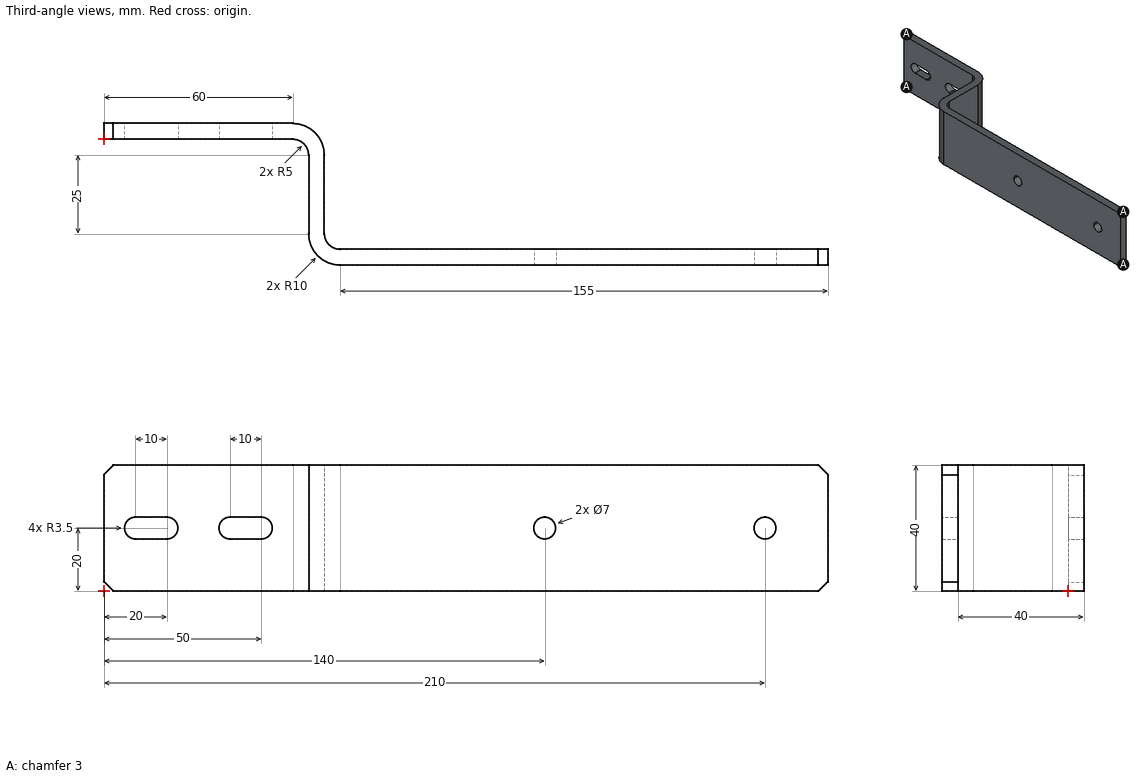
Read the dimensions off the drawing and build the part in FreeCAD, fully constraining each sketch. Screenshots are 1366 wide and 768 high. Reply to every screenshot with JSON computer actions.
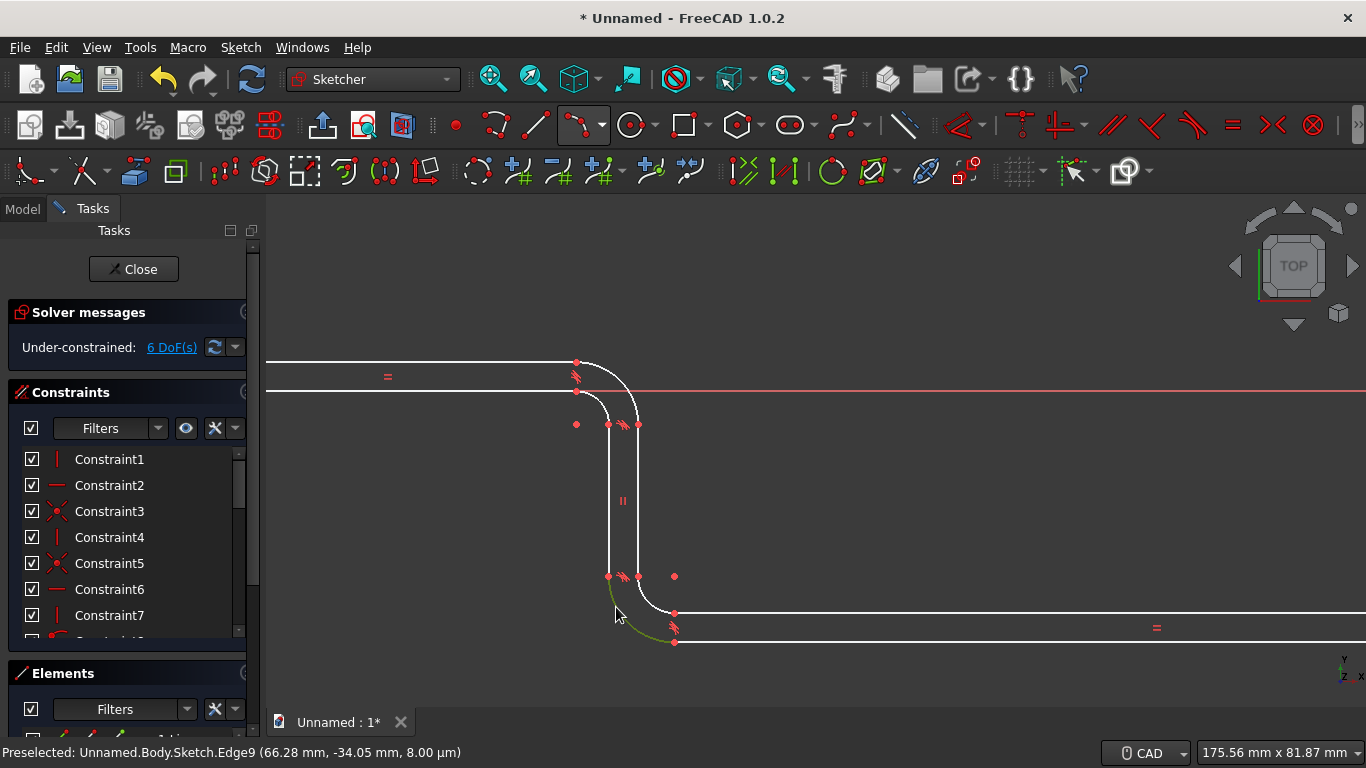
{"action": "left_click", "coordinate": [604, 369]}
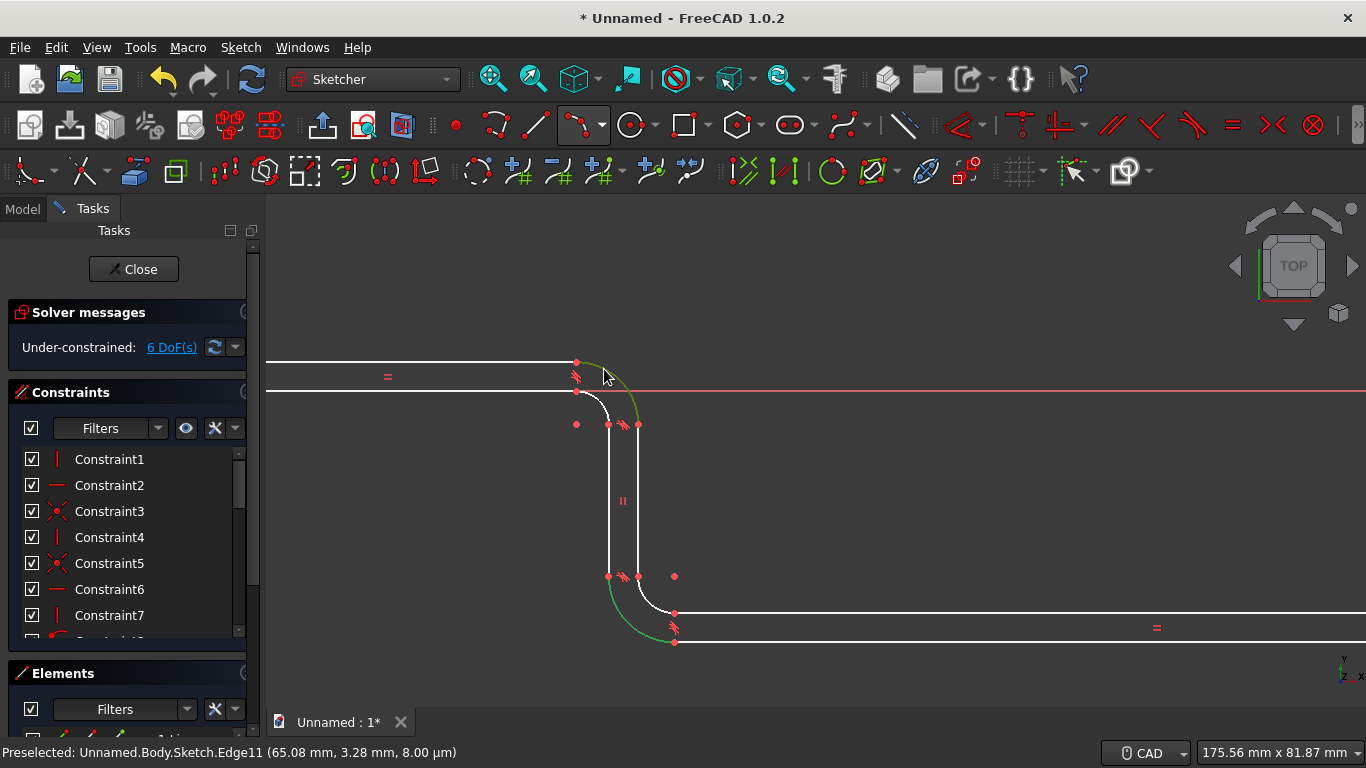
{"action": "left_click", "coordinate": [1234, 126]}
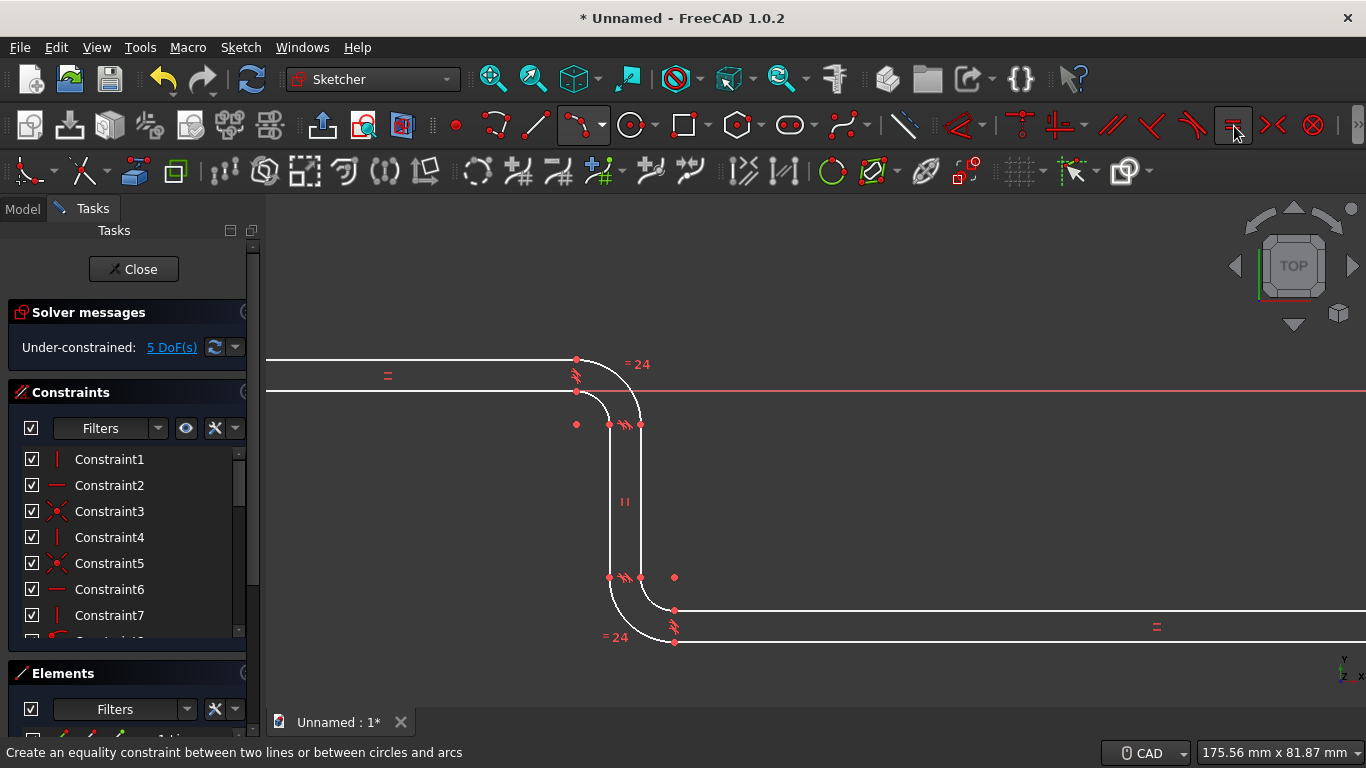
{"action": "left_click", "coordinate": [617, 607]}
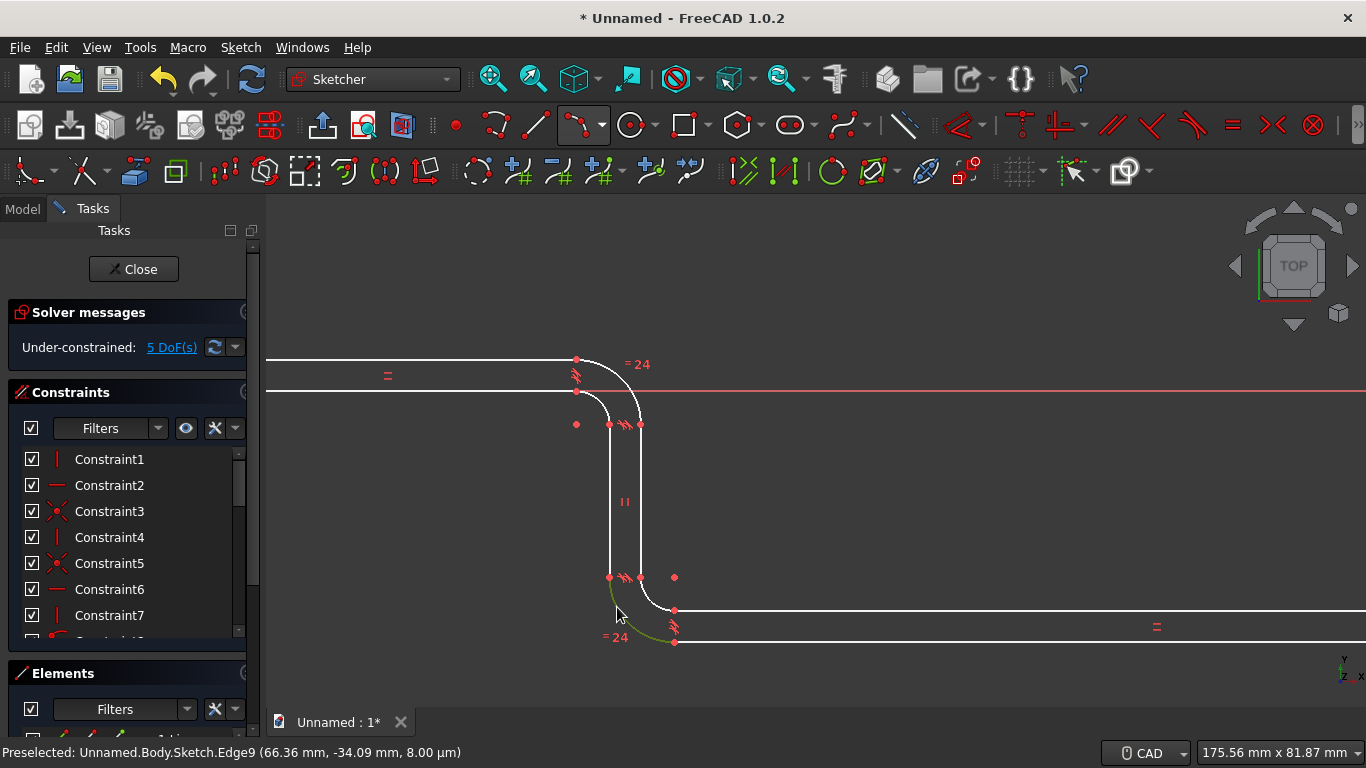
{"action": "left_click", "coordinate": [984, 126]}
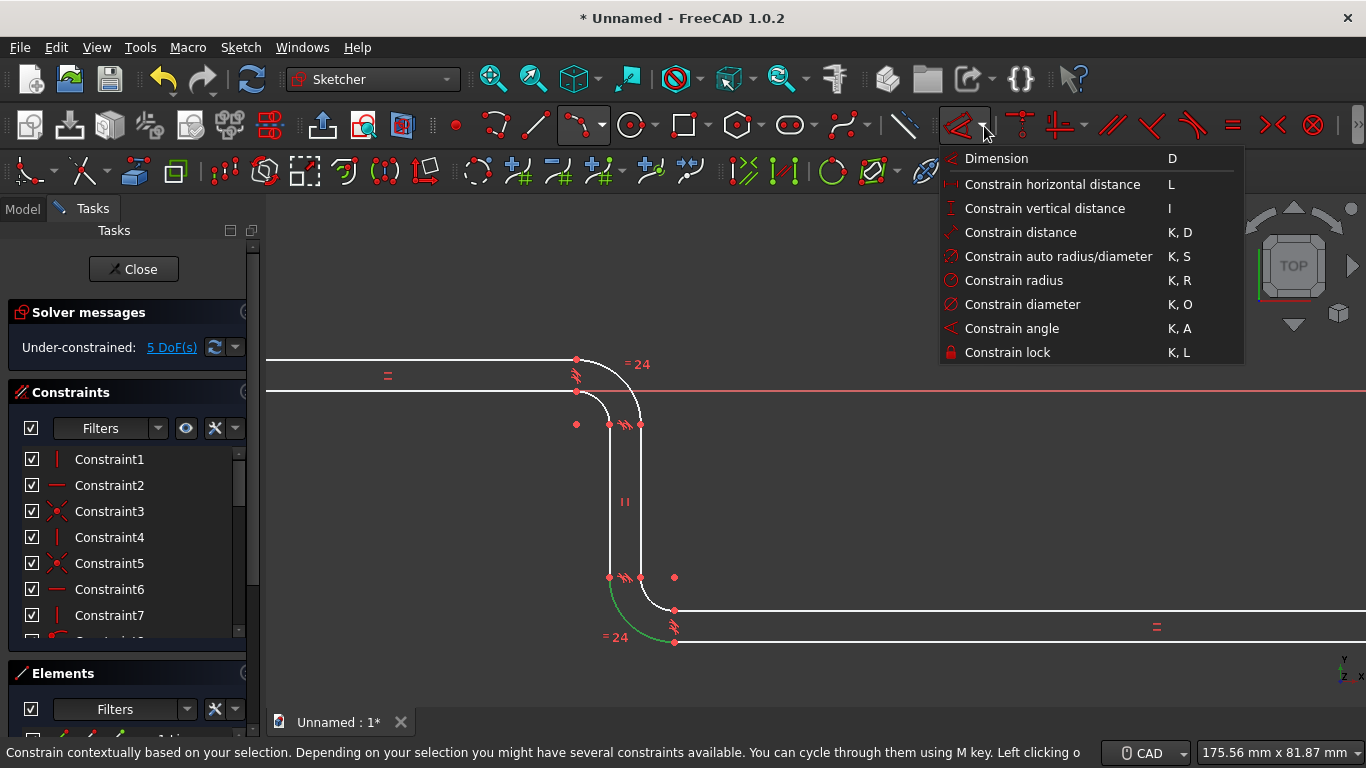
{"action": "left_click", "coordinate": [1092, 280]}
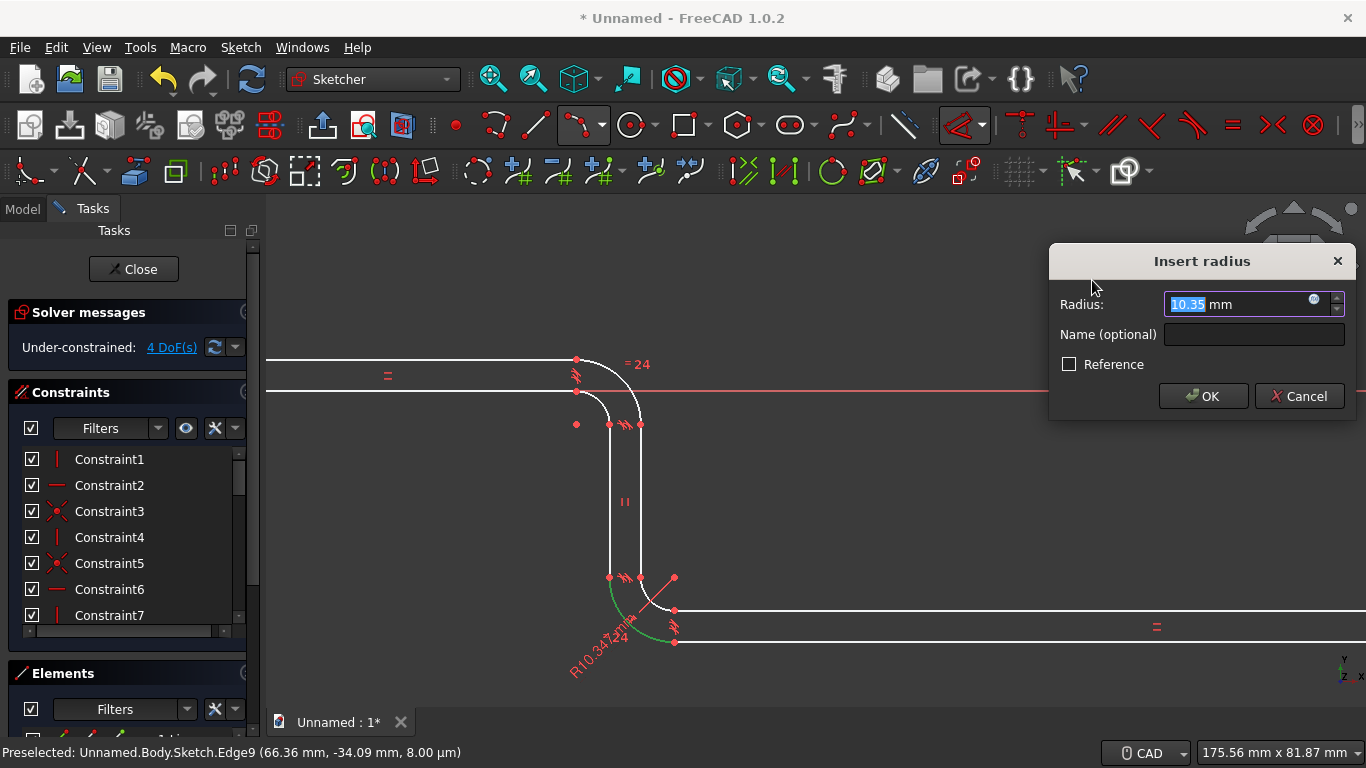
{"action": "type", "text": "10"}
{"action": "key", "text": "Return"}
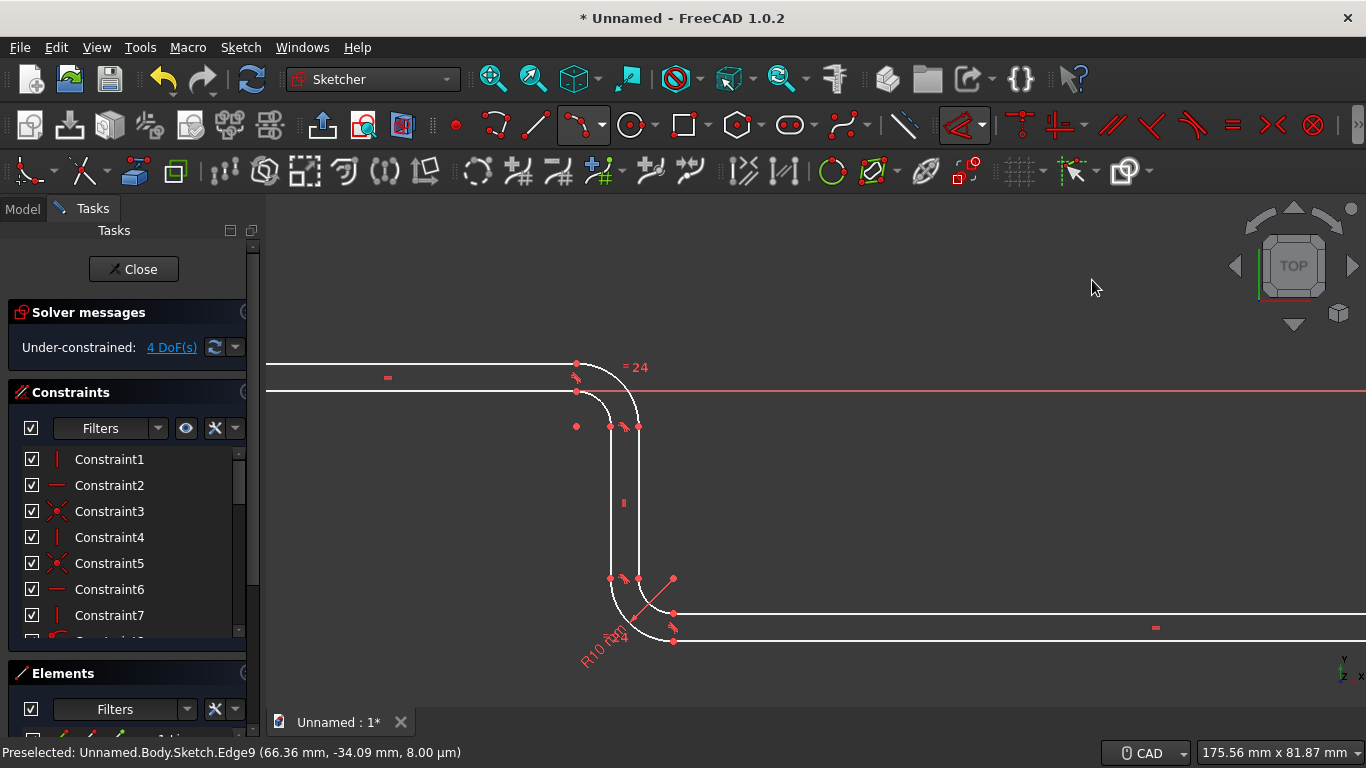
{"action": "scroll", "coordinate": [643, 595], "scroll_direction": "up", "scroll_amount": 2}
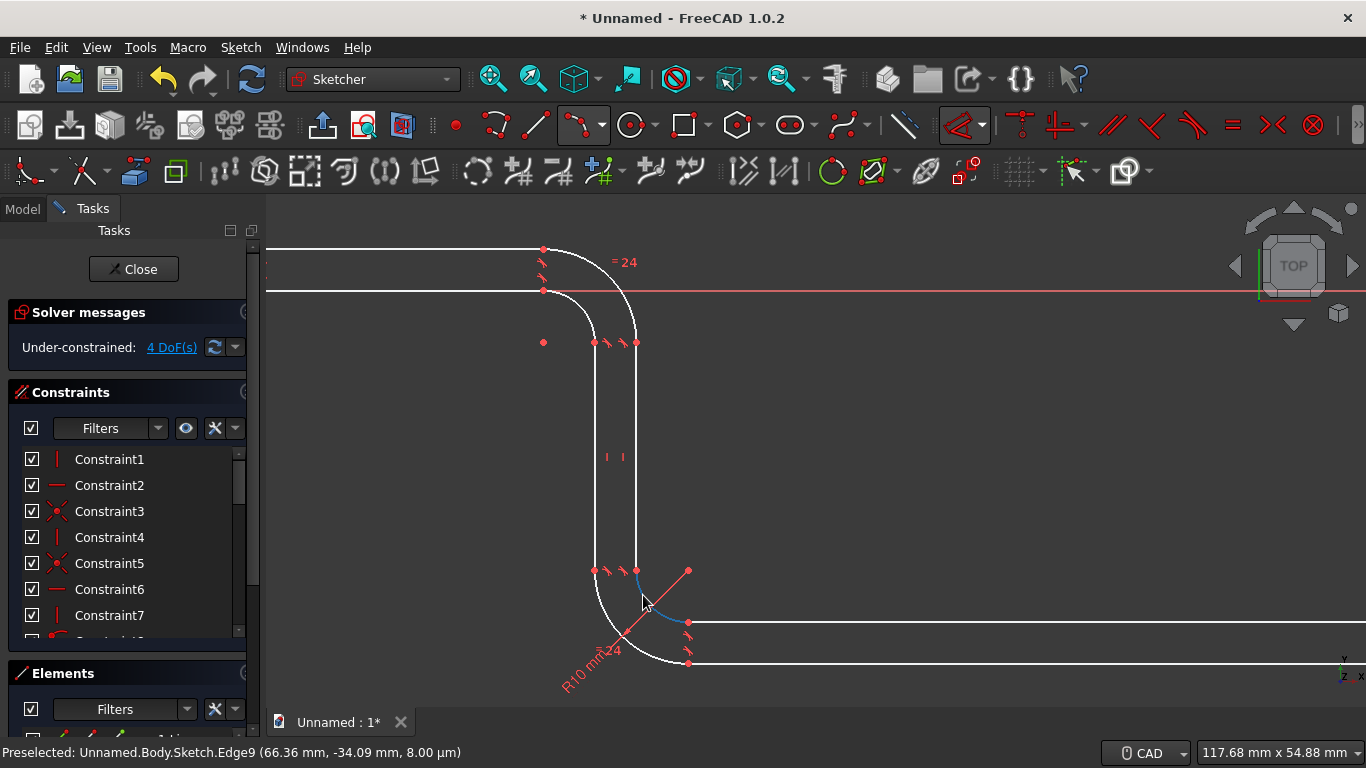
{"action": "left_click", "coordinate": [642, 594]}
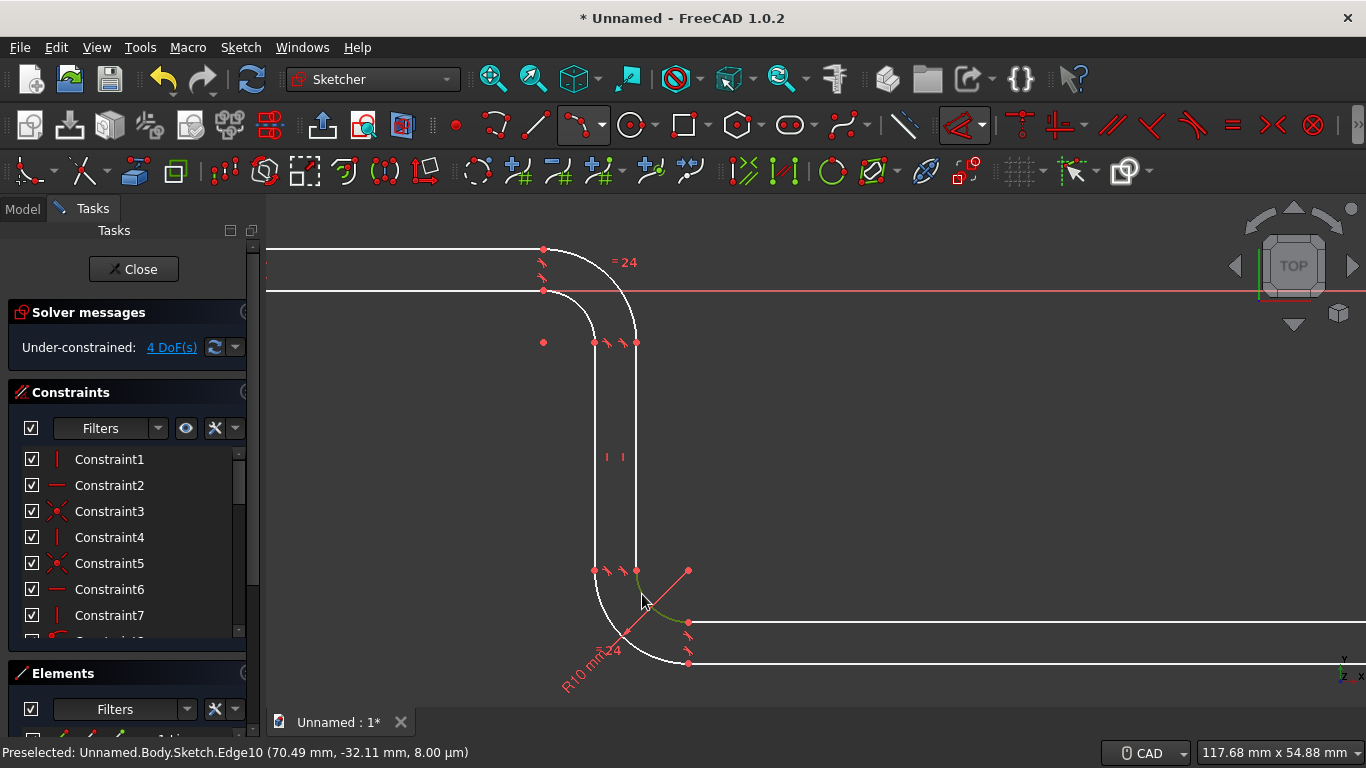
{"action": "left_click", "coordinate": [984, 126]}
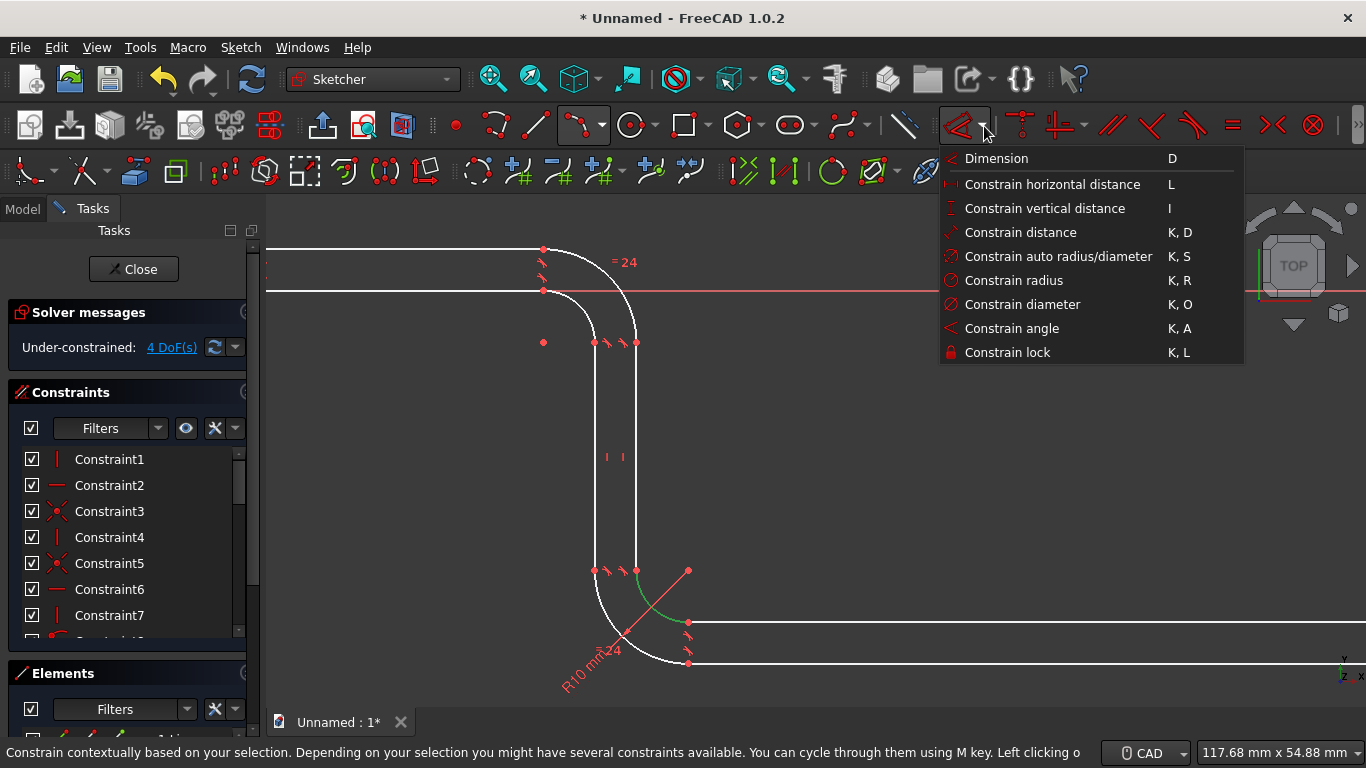
{"action": "left_click", "coordinate": [1092, 280]}